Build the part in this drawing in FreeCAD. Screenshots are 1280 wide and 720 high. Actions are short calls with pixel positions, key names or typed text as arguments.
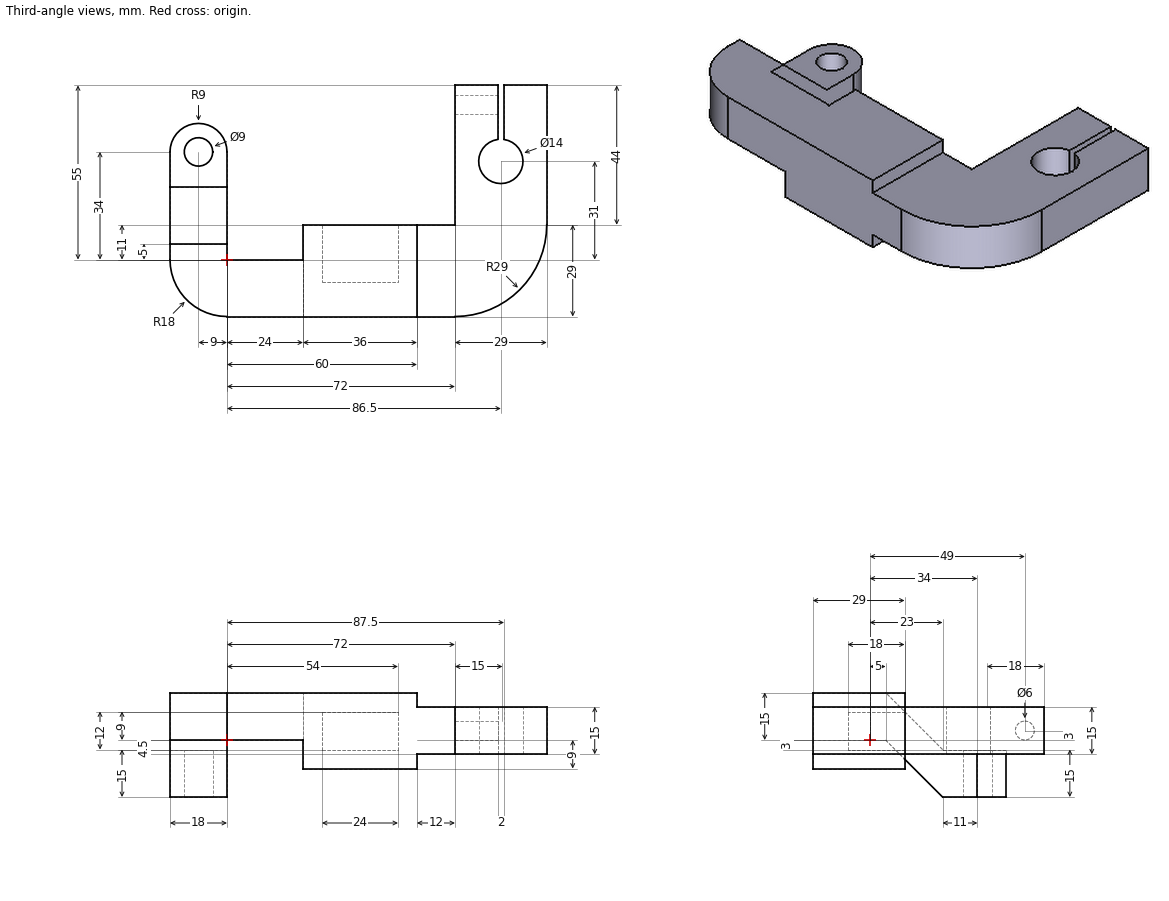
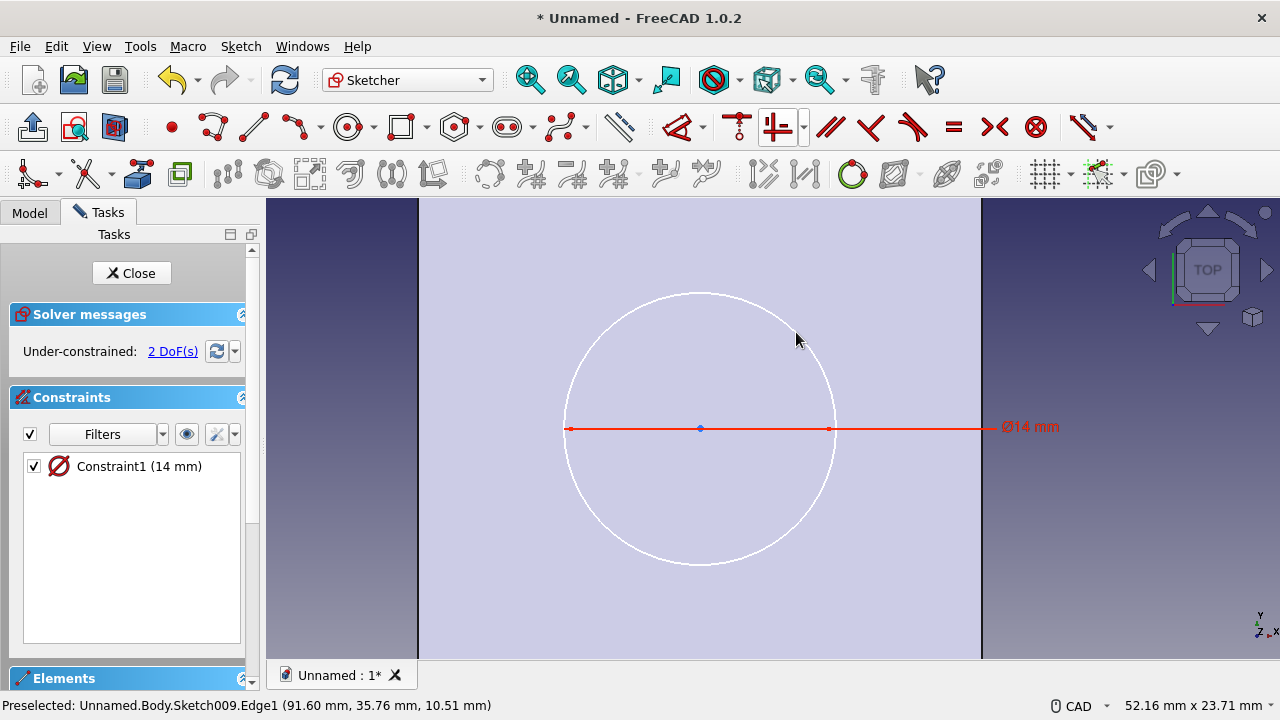
click(676, 128)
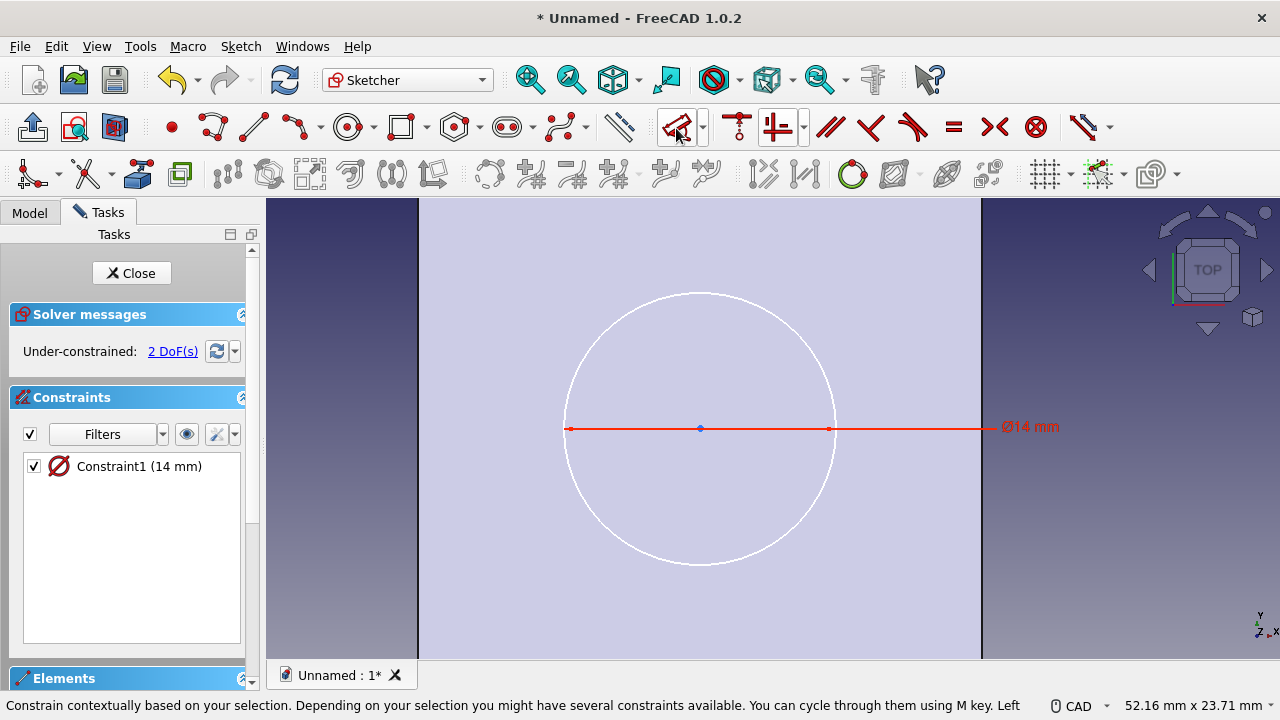
click(700, 429)
click(734, 530)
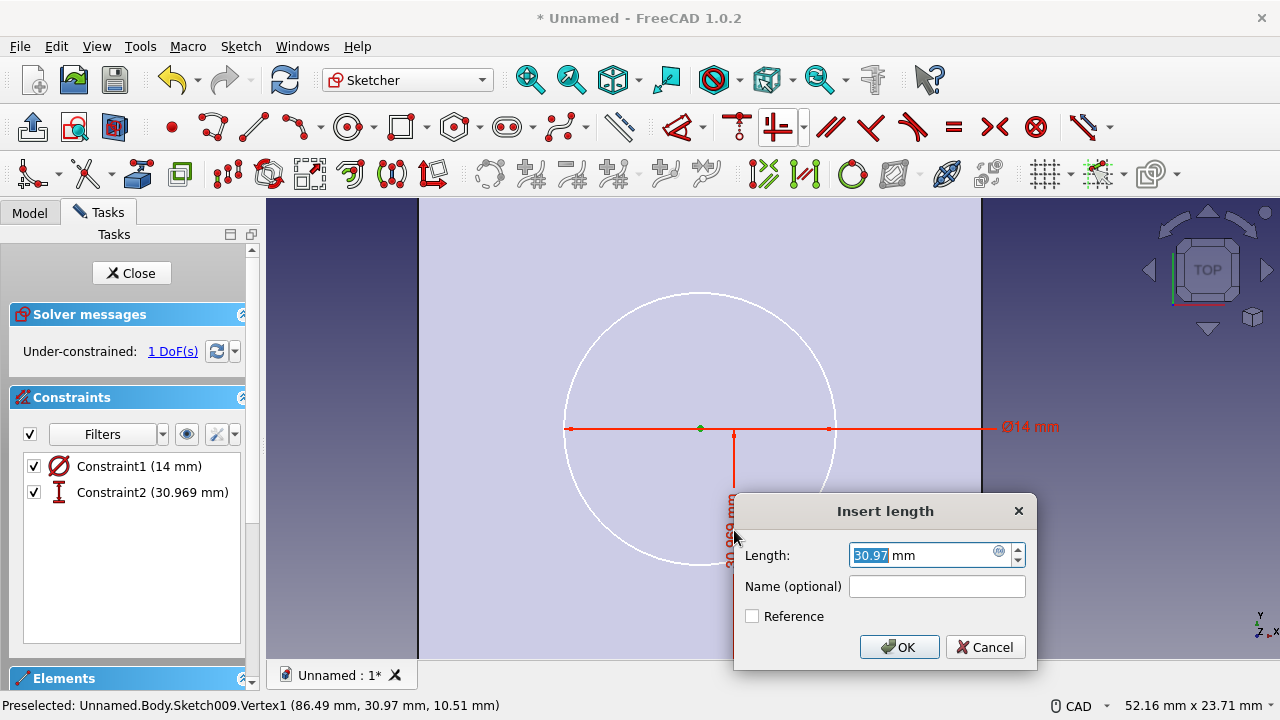
text(31)
key(Return)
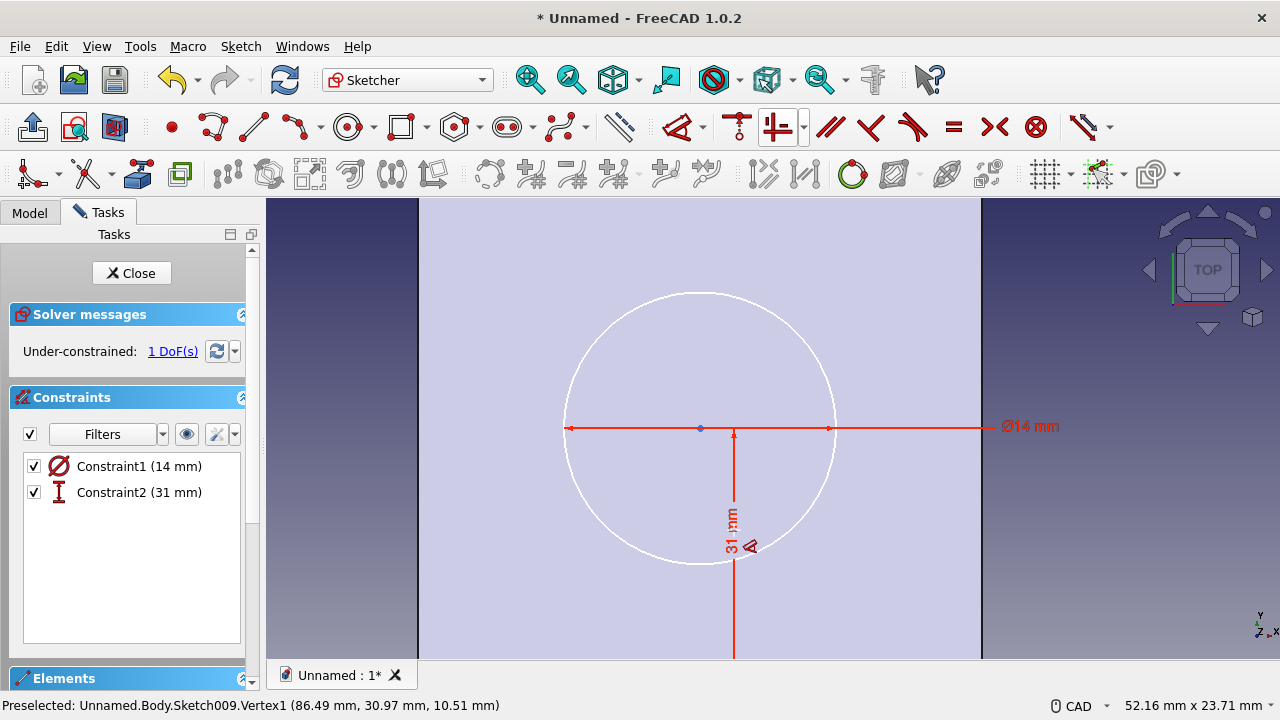
click(700, 428)
click(497, 394)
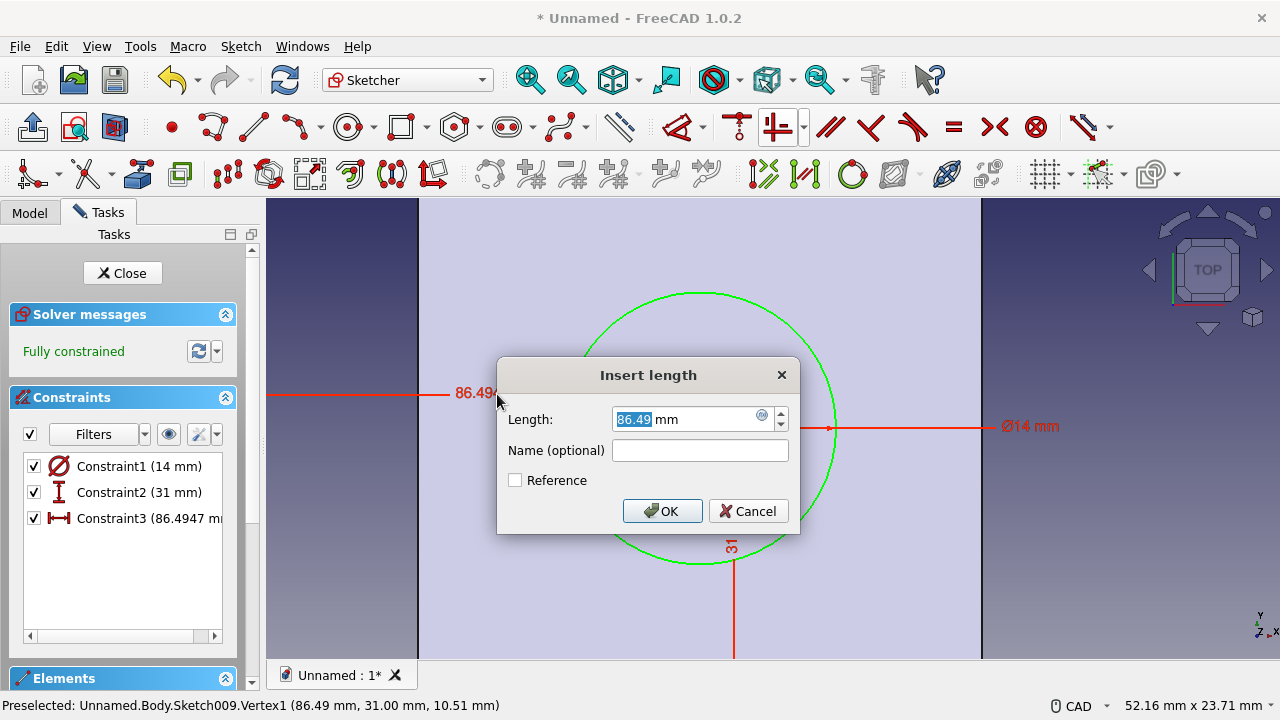
text(86.5)
key(Return)
key(Escape)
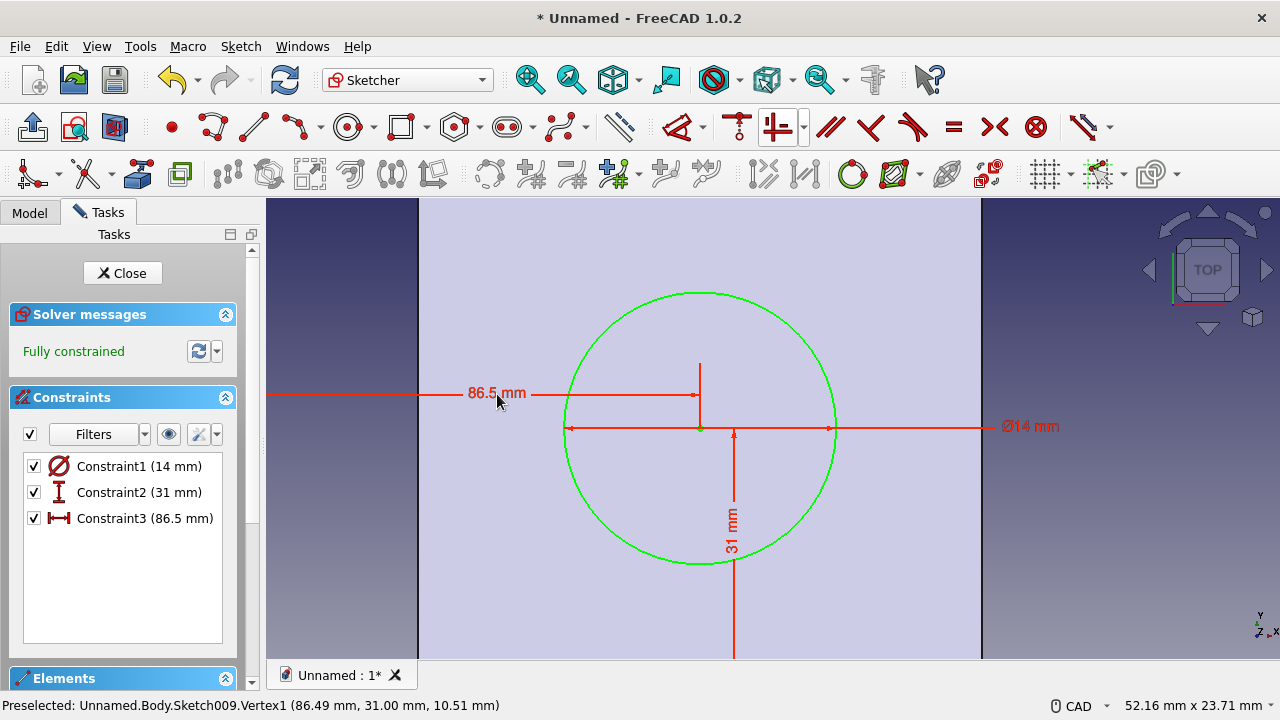
click(123, 273)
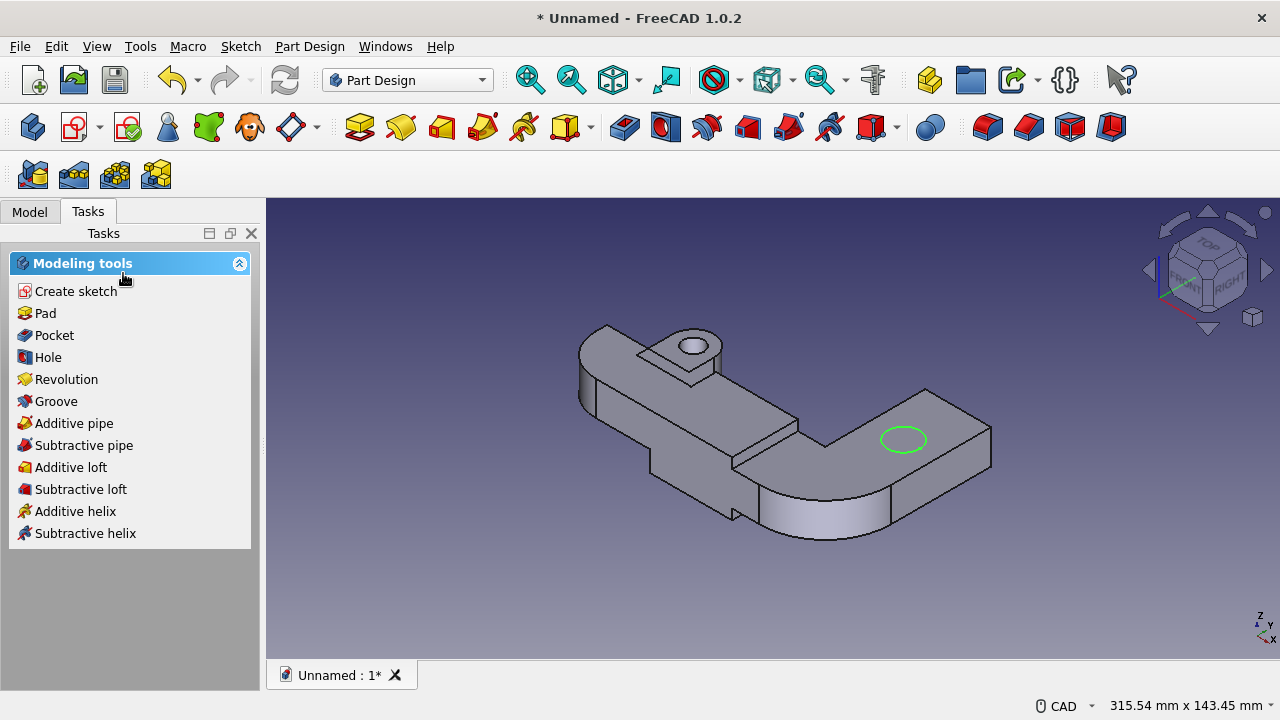
click(625, 128)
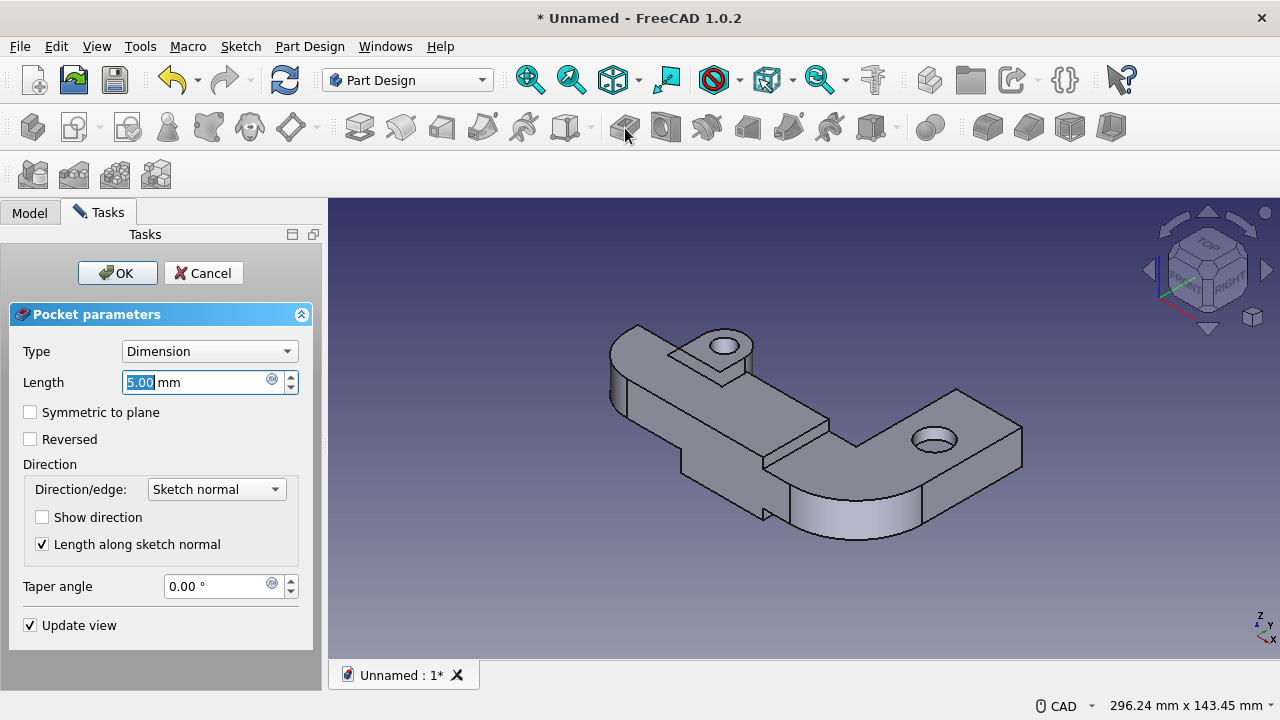
text(15)
key(Tab)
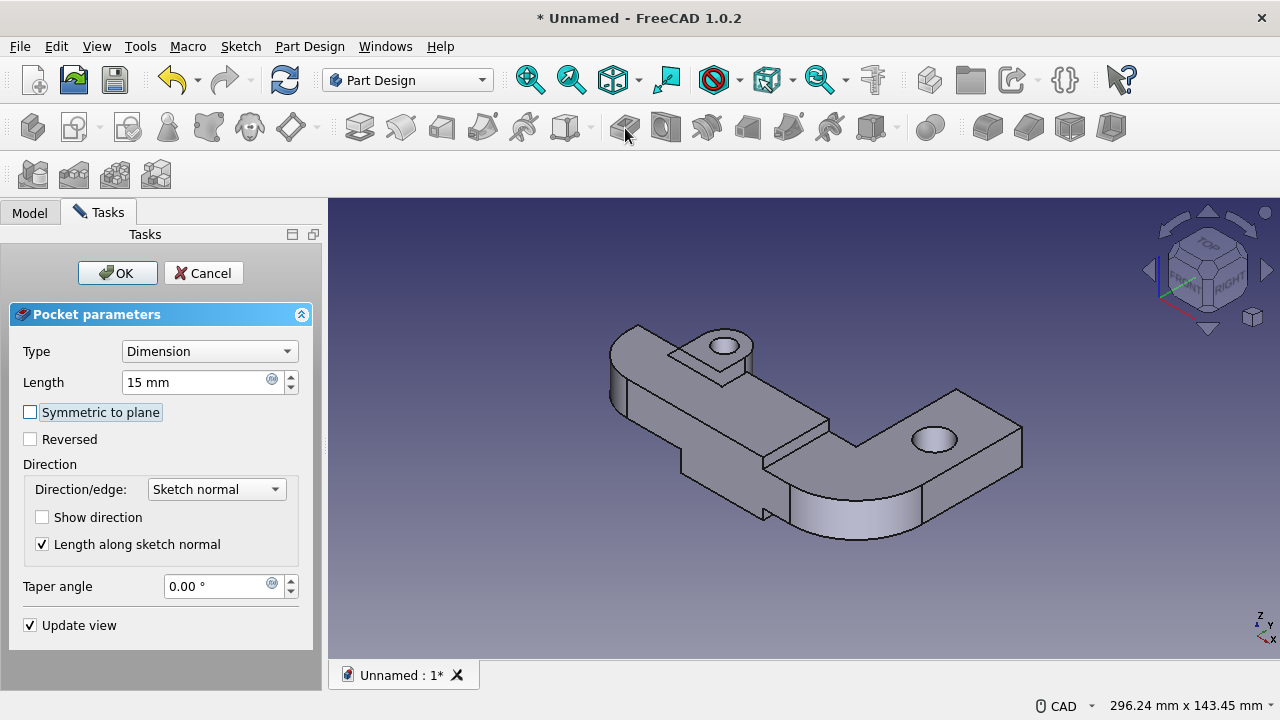
click(118, 273)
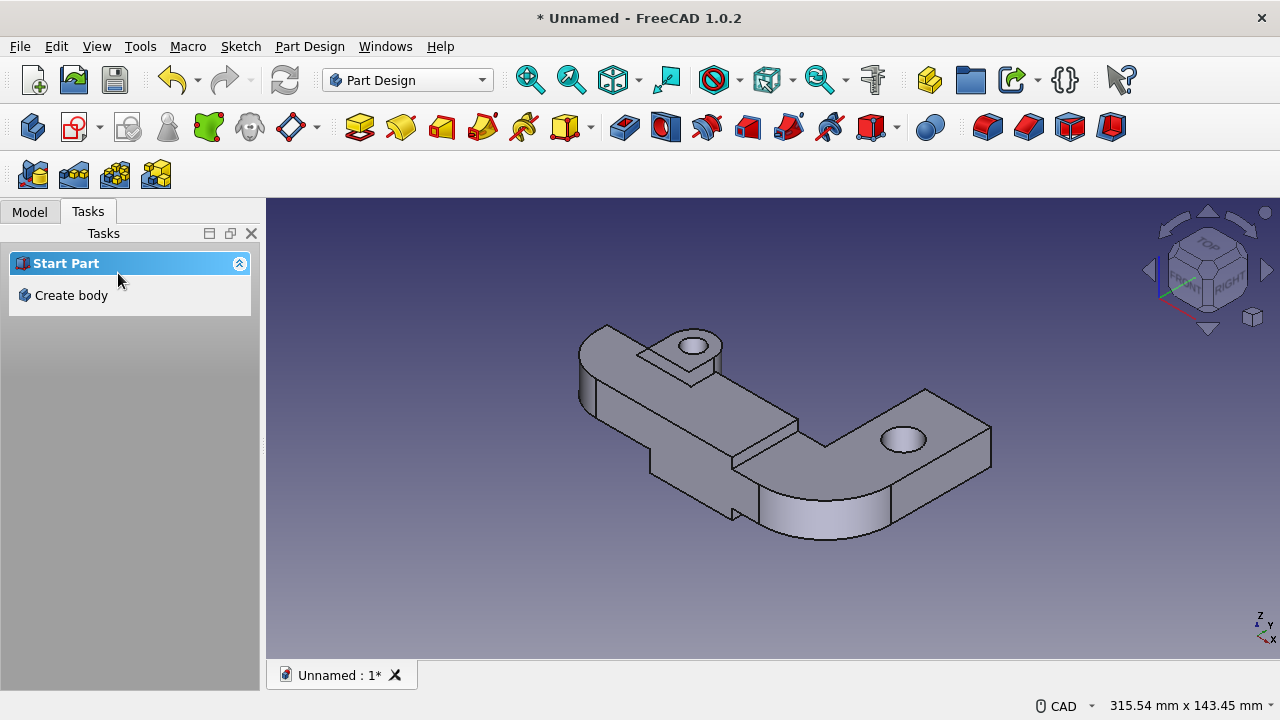
key(4)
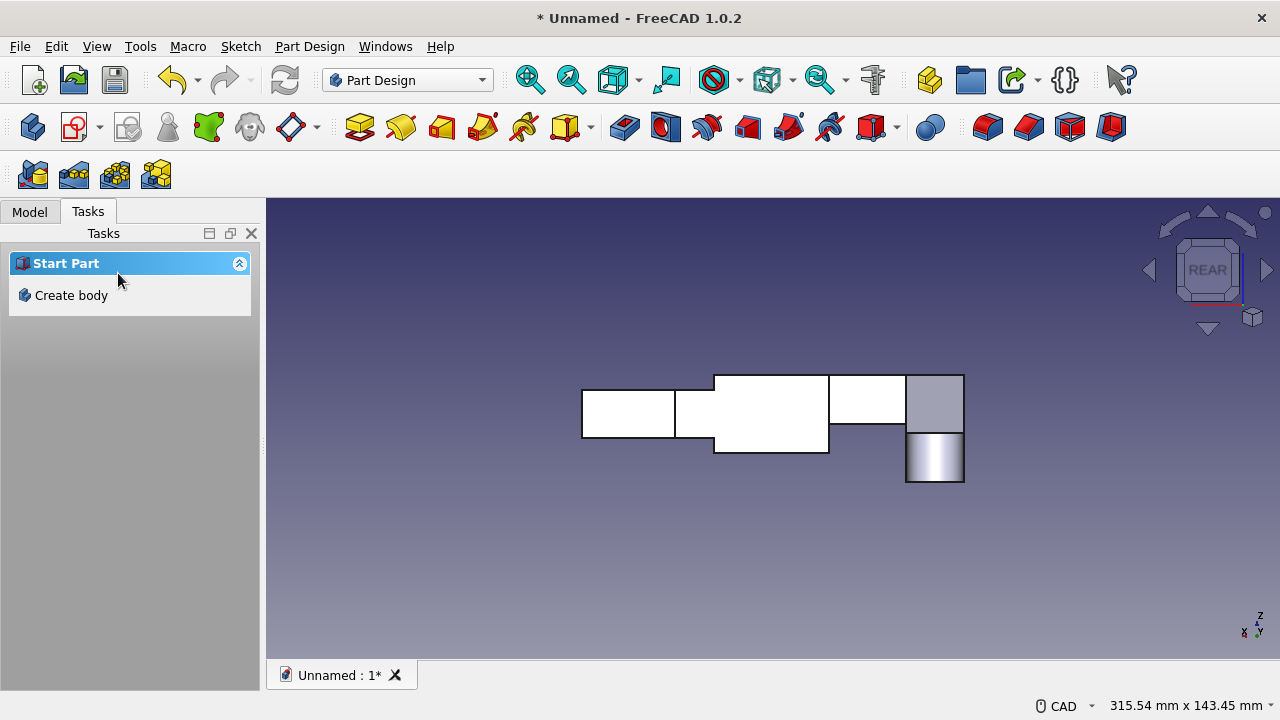
click(531, 80)